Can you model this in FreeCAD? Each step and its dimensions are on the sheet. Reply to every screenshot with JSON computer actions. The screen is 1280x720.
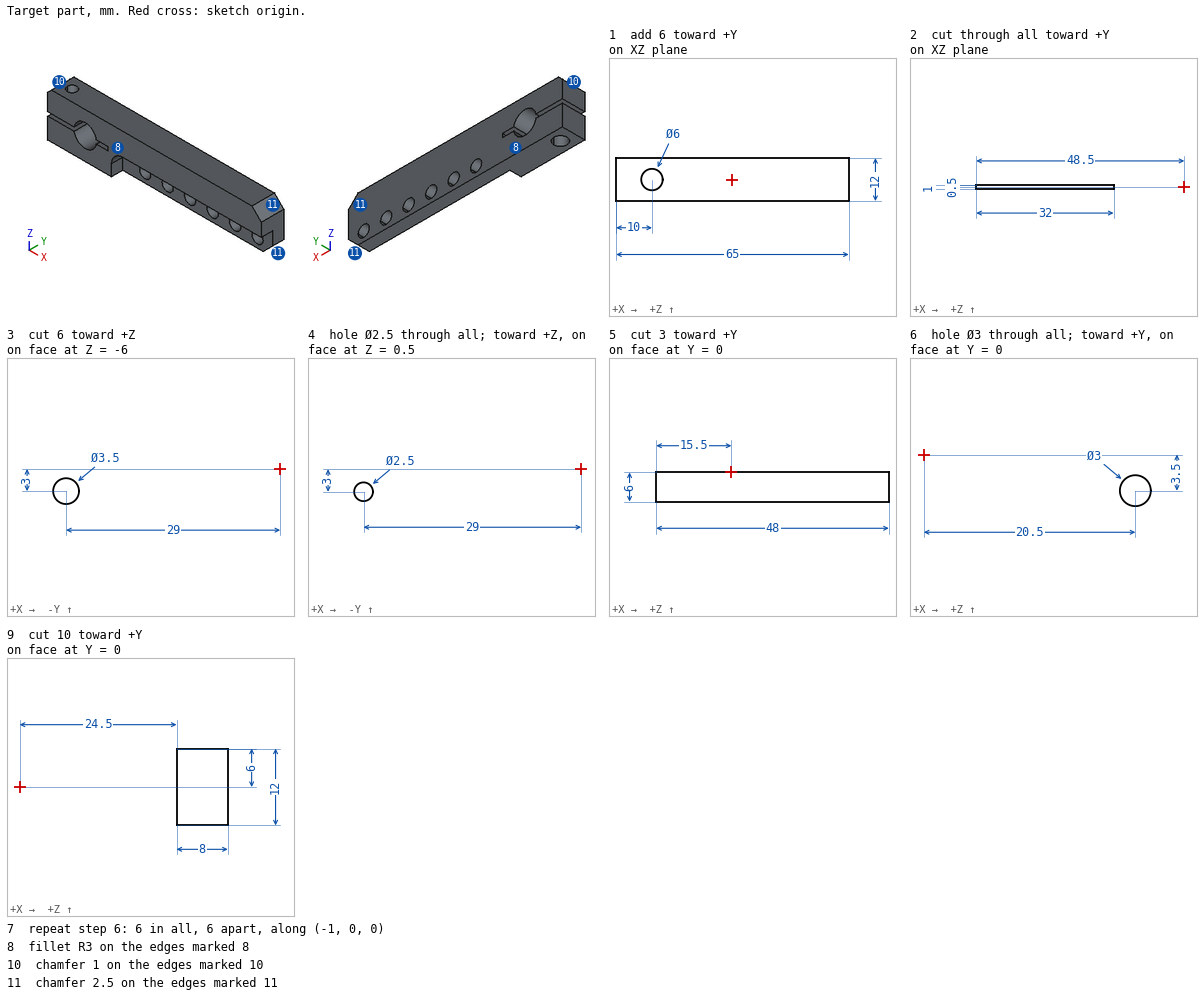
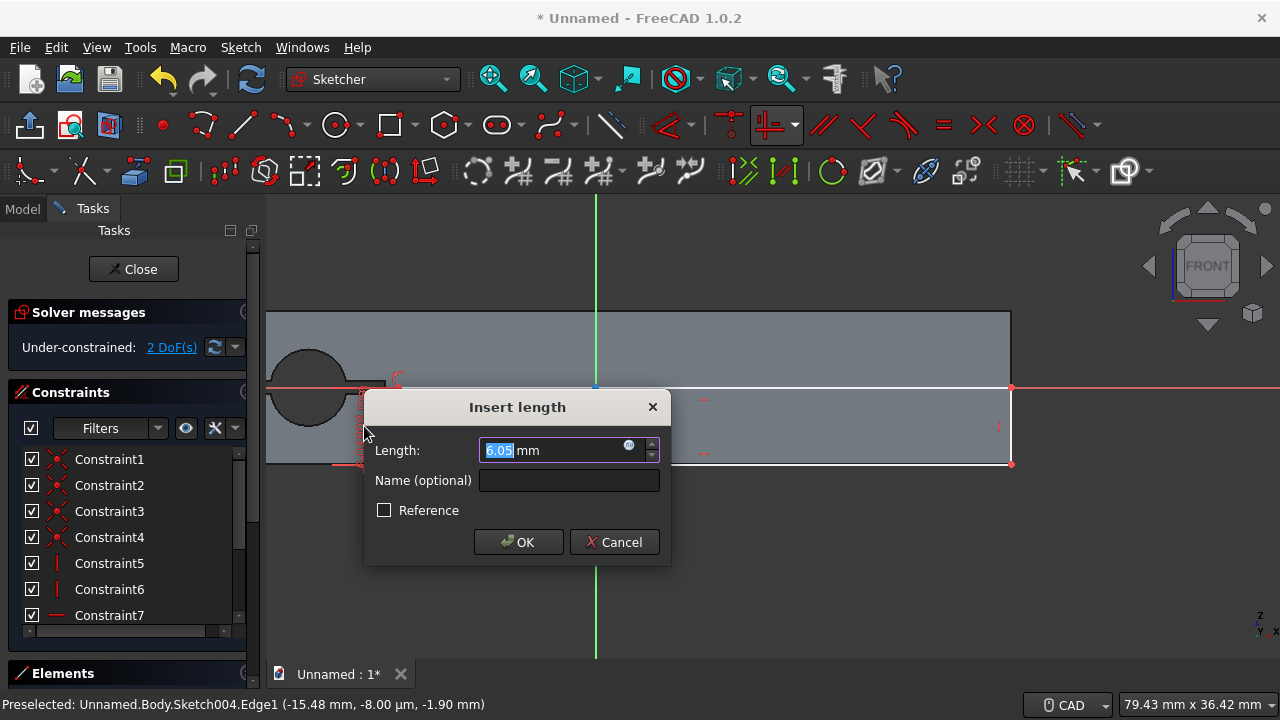
{"action": "type", "text": "6"}
{"action": "key", "text": "Return"}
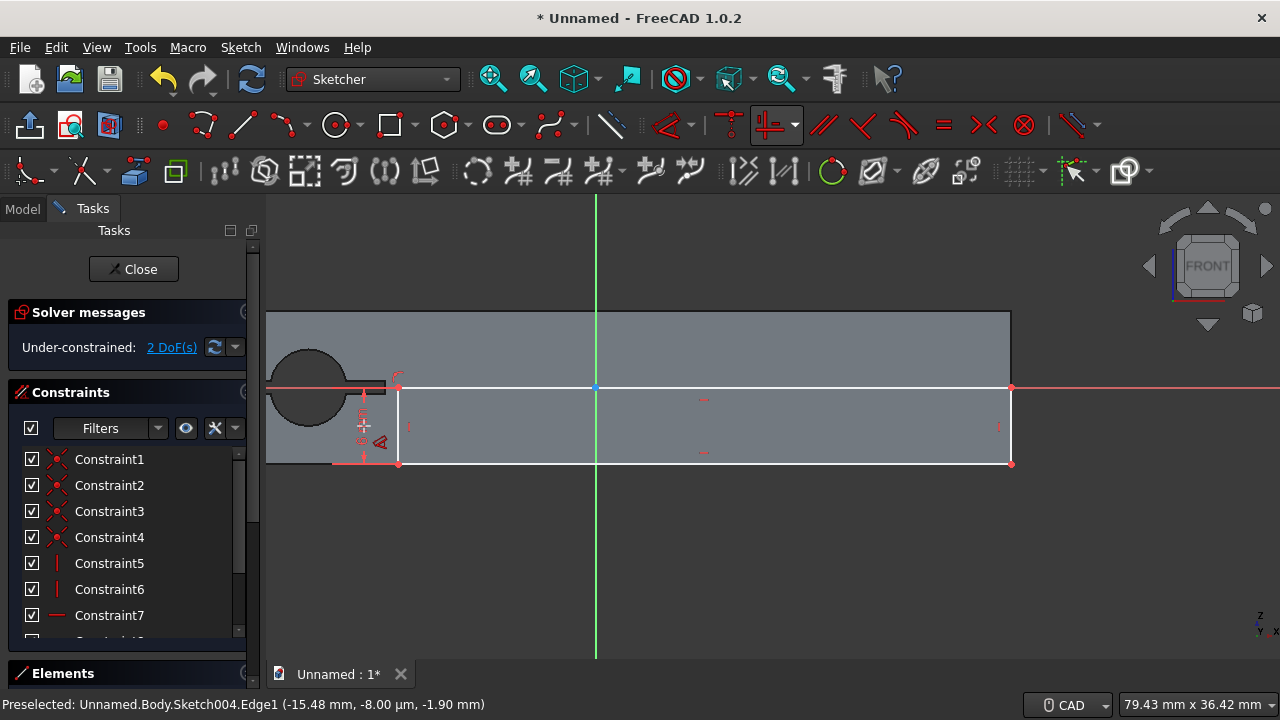
{"action": "left_click", "coordinate": [582, 464]}
{"action": "left_click", "coordinate": [704, 498]}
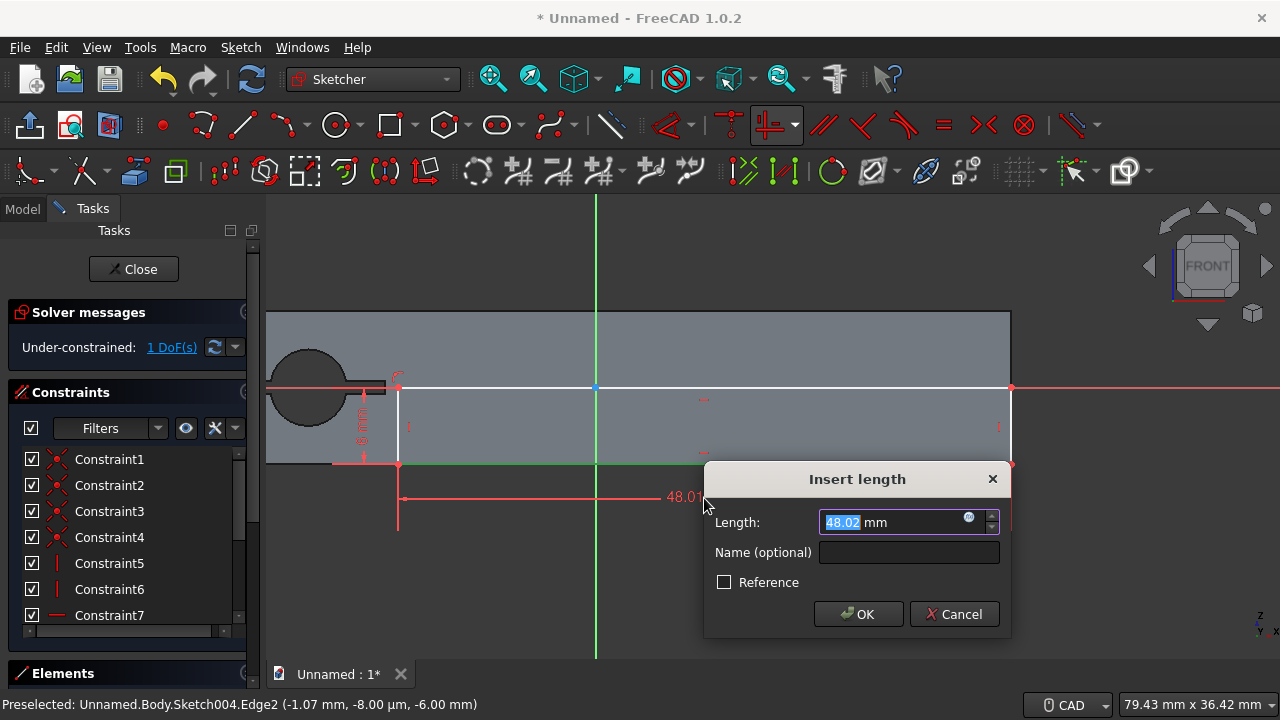
{"action": "type", "text": "48"}
{"action": "key", "text": "Return"}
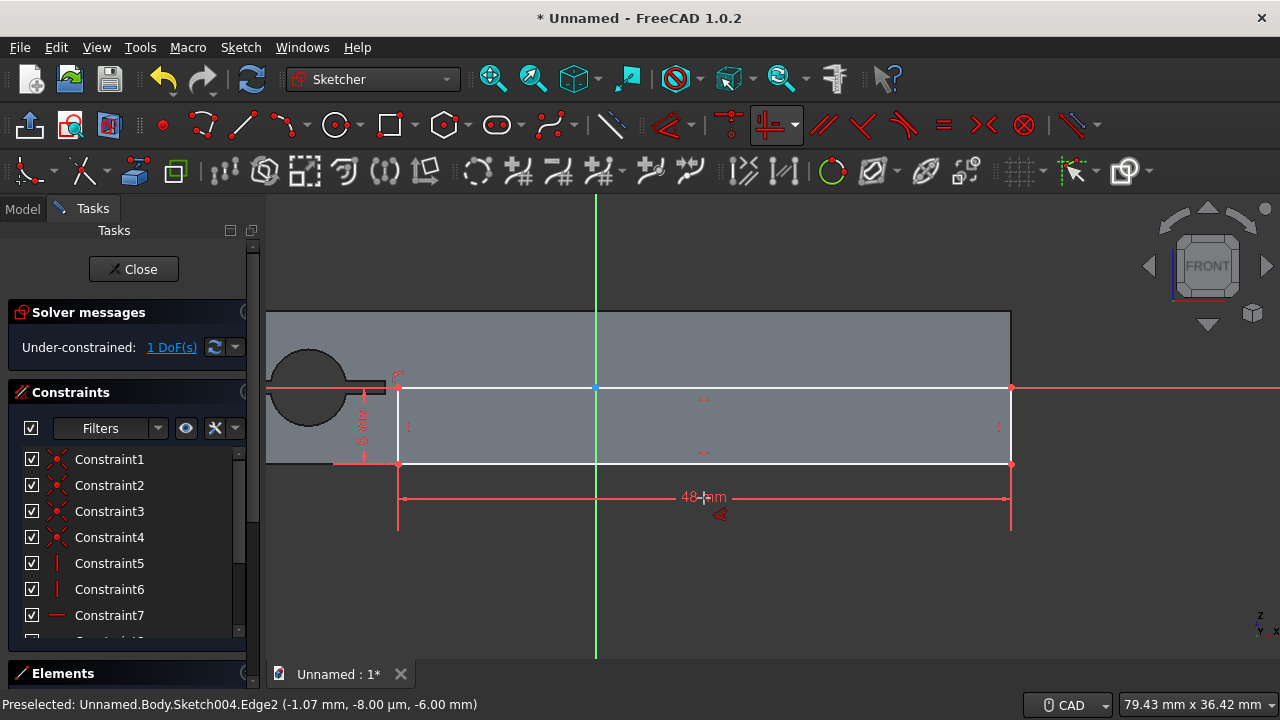
{"action": "left_click", "coordinate": [398, 388]}
{"action": "left_click", "coordinate": [497, 354]}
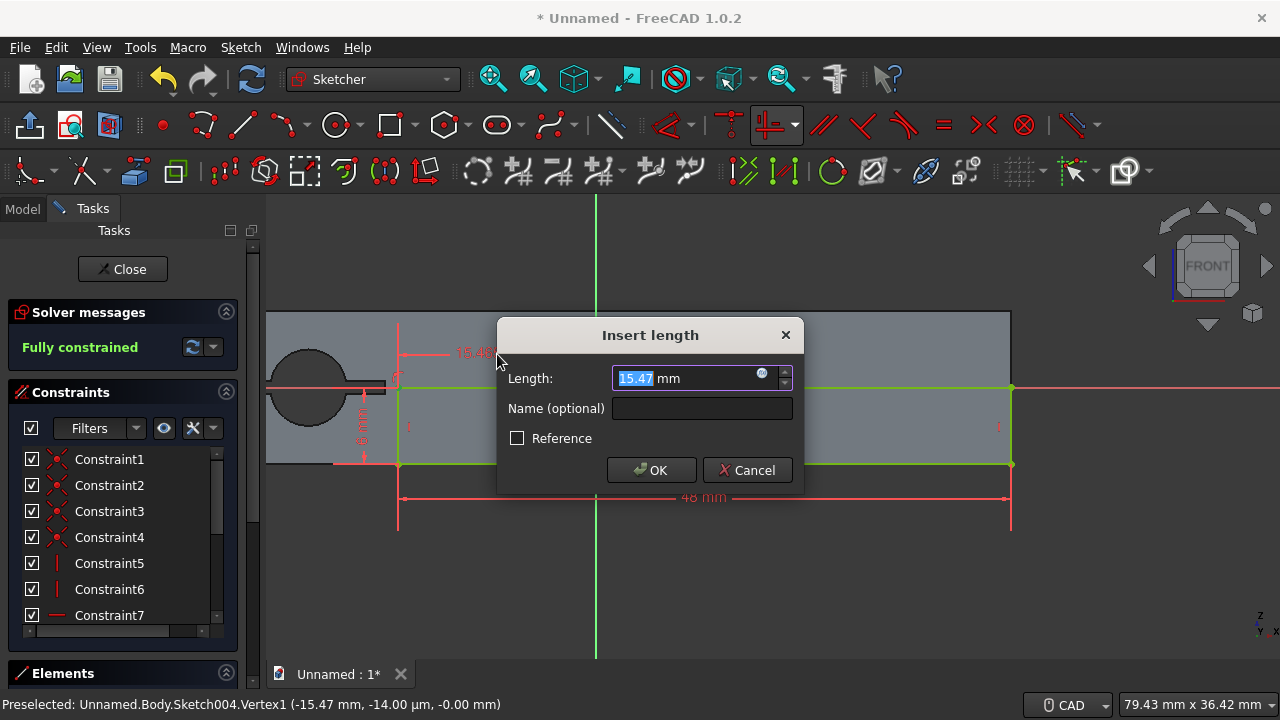
{"action": "type", "text": "15.5"}
{"action": "key", "text": "Return"}
{"action": "key", "text": "Escape"}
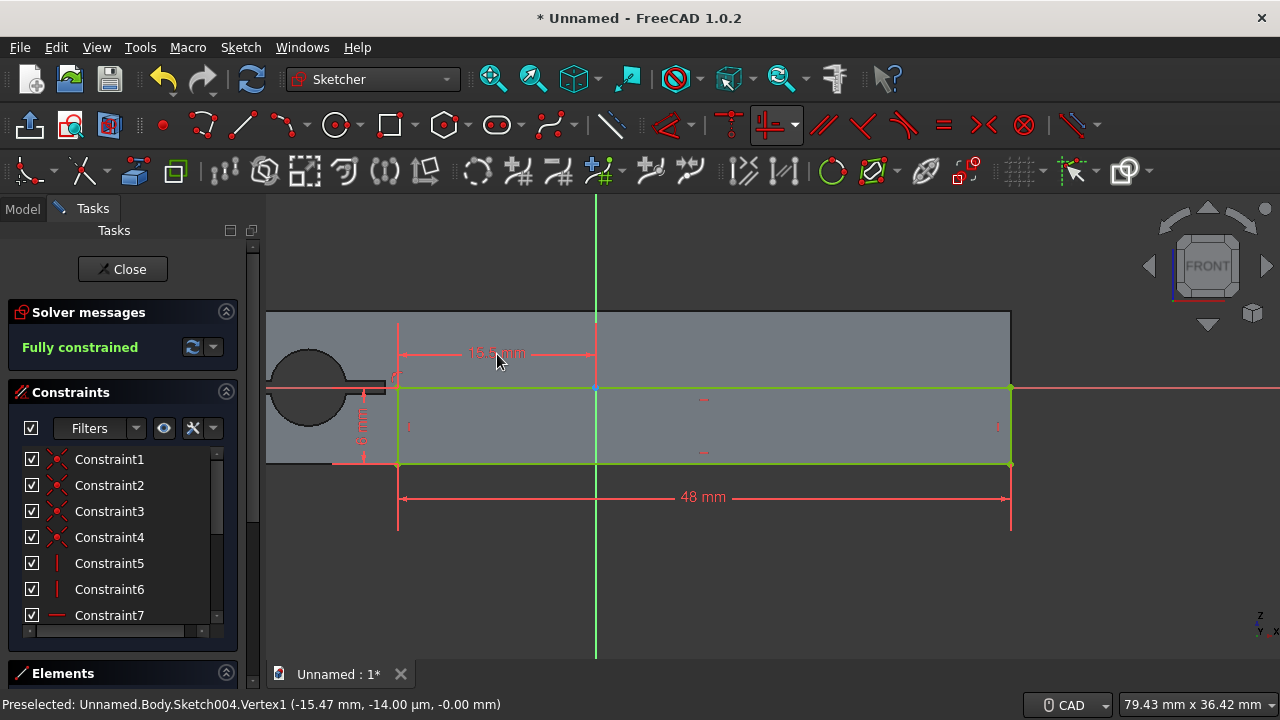
{"action": "left_click", "coordinate": [123, 269]}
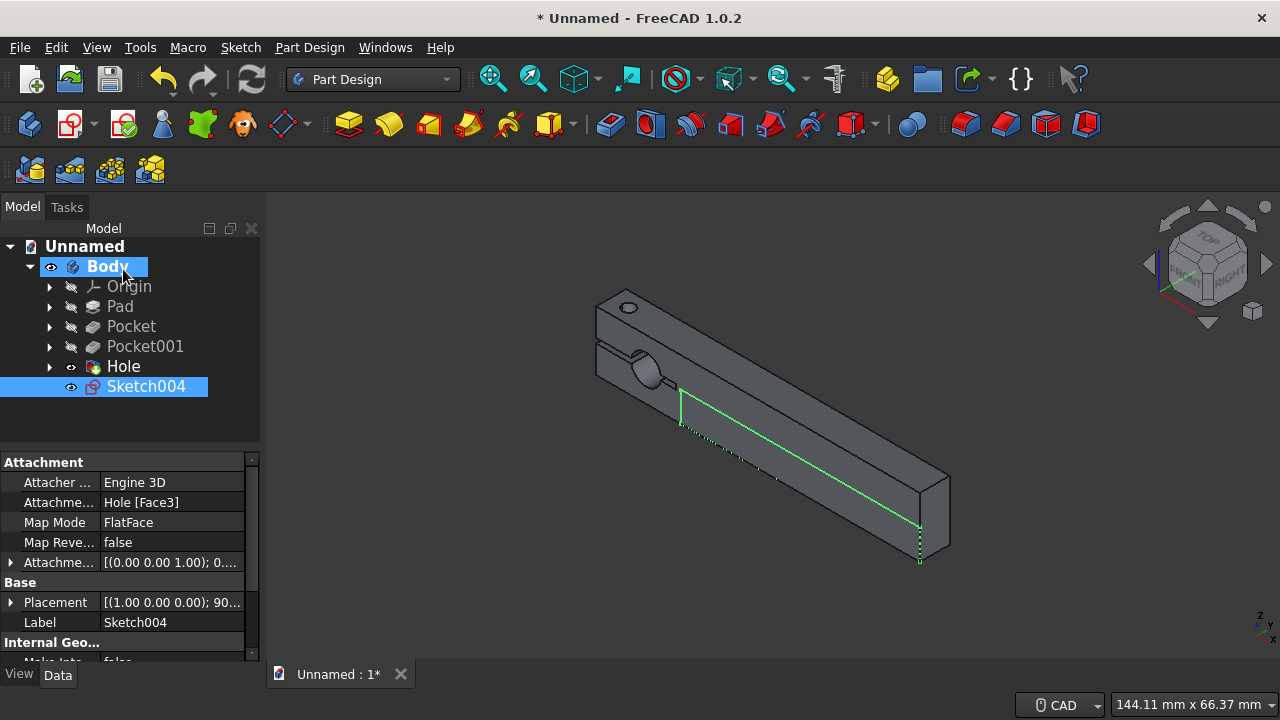
{"action": "left_click", "coordinate": [612, 124]}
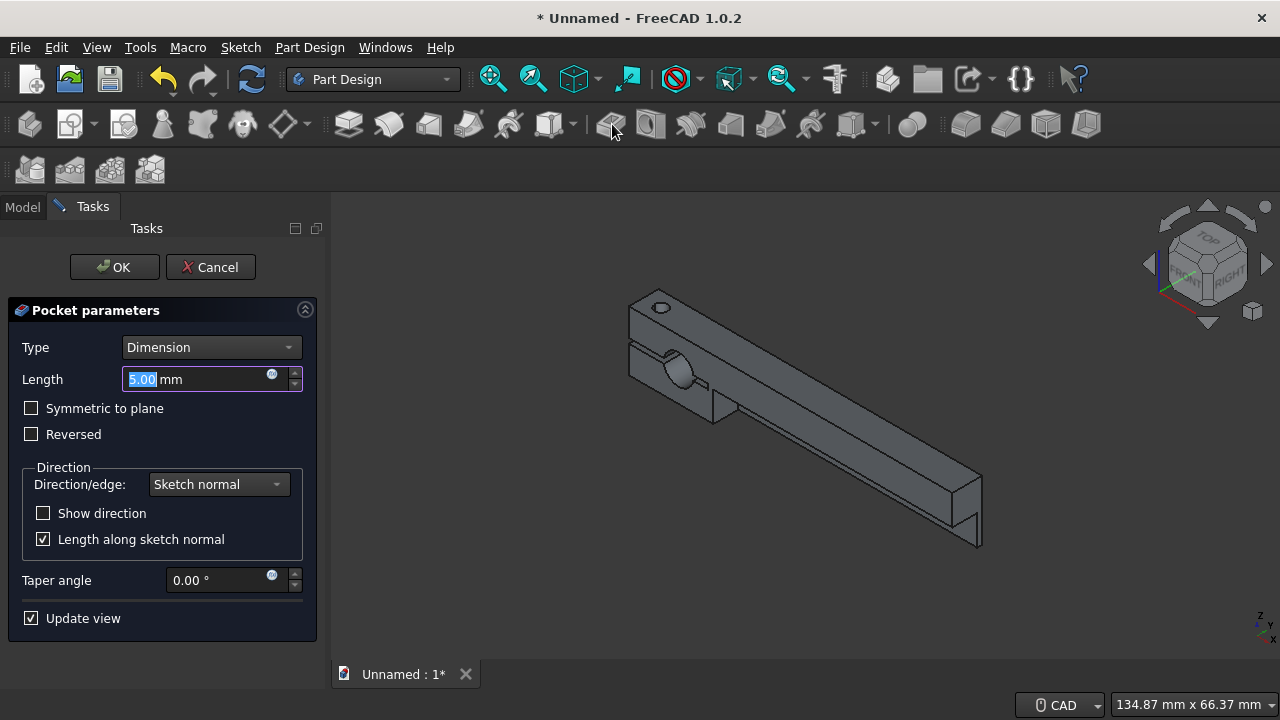
{"action": "type", "text": "3"}
{"action": "key", "text": "Tab"}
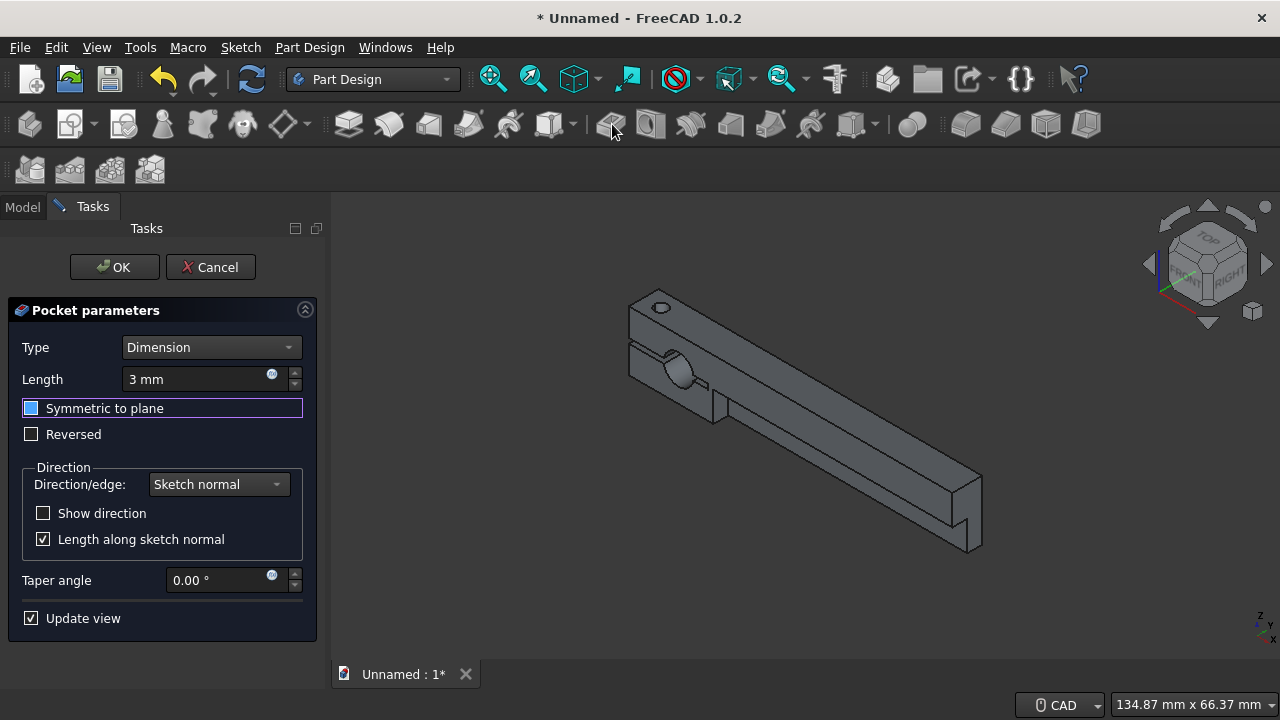
{"action": "left_click", "coordinate": [115, 267]}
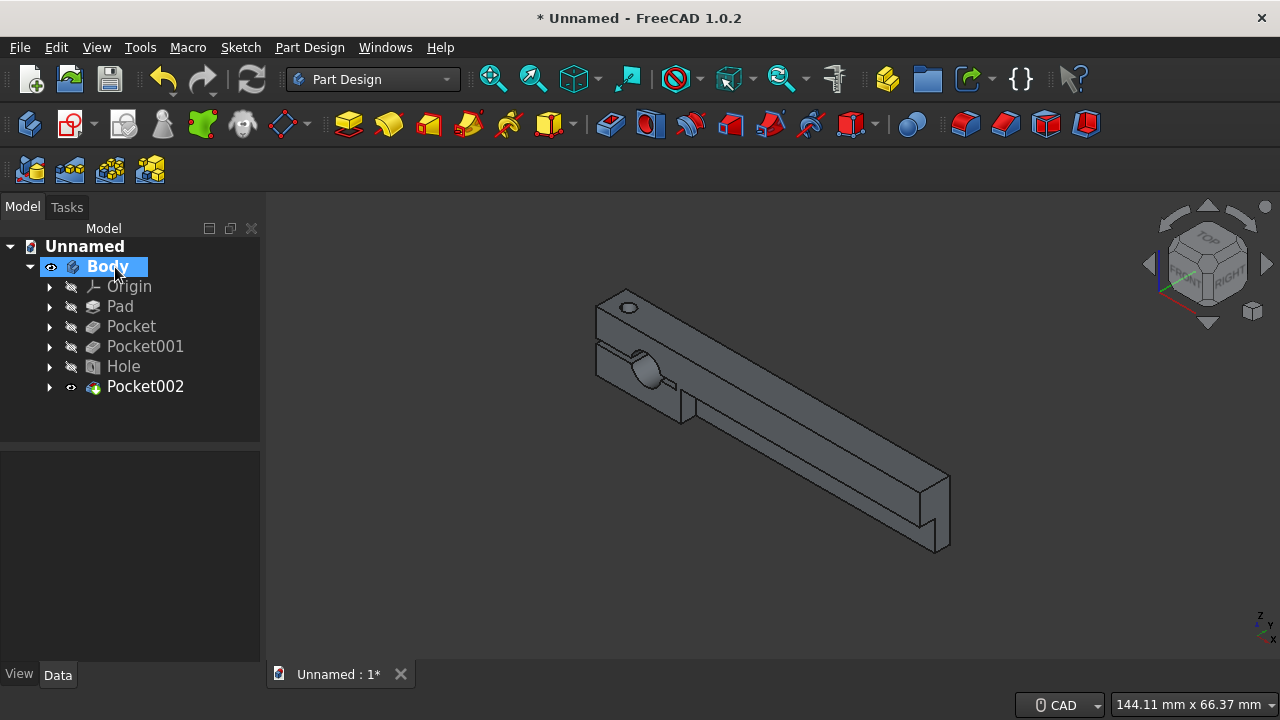
{"action": "left_click", "coordinate": [619, 373]}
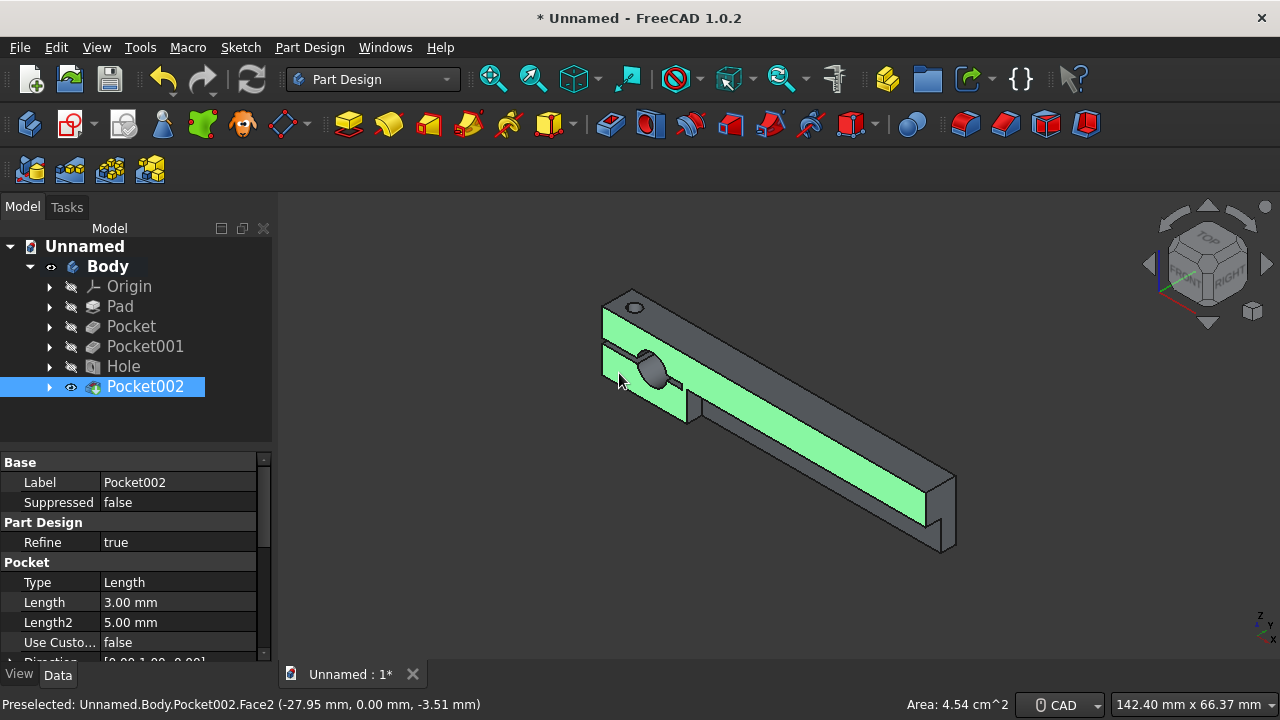
{"action": "left_click", "coordinate": [70, 124]}